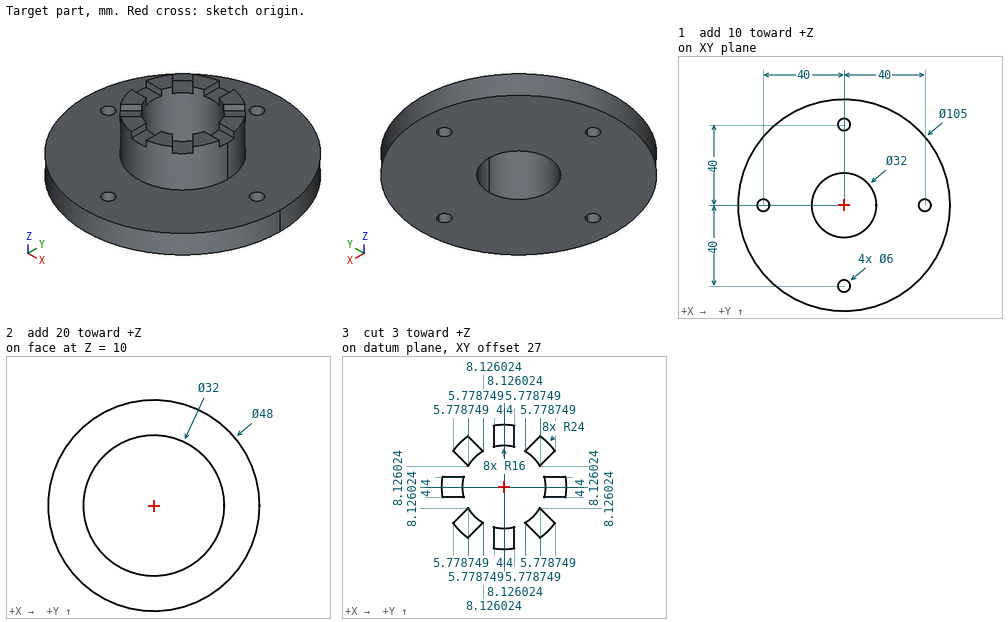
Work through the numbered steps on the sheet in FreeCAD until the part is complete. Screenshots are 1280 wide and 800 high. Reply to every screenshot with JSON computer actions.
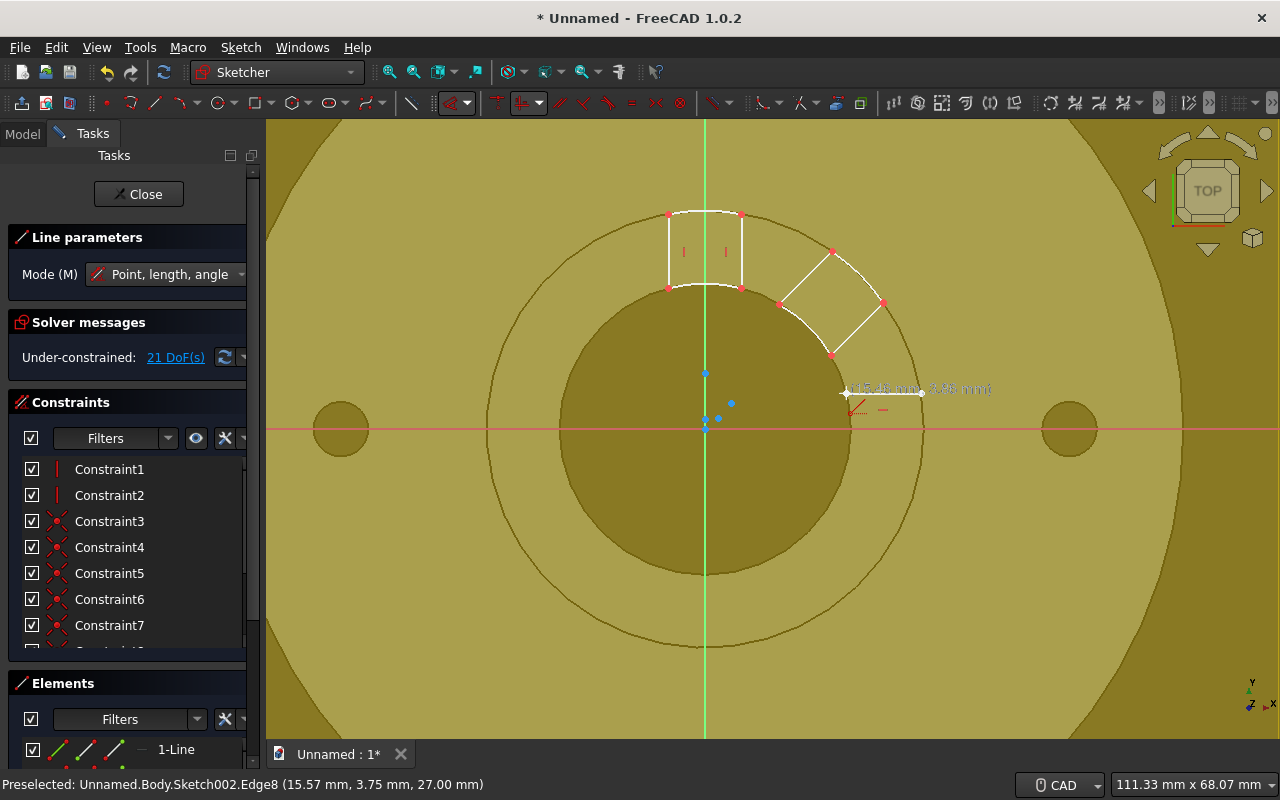
{"action": "left_click", "coordinate": [846, 466]}
{"action": "left_click", "coordinate": [921, 466]}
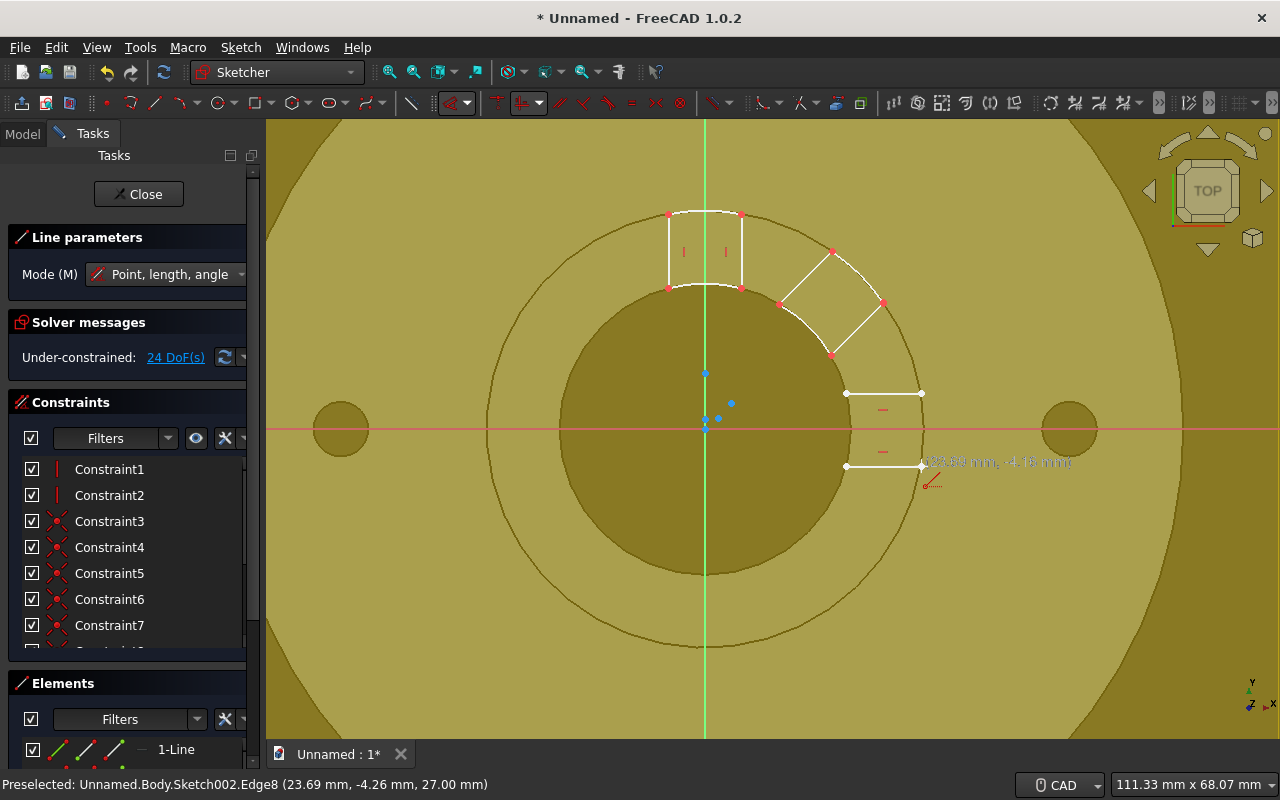
{"action": "left_click", "coordinate": [180, 104]}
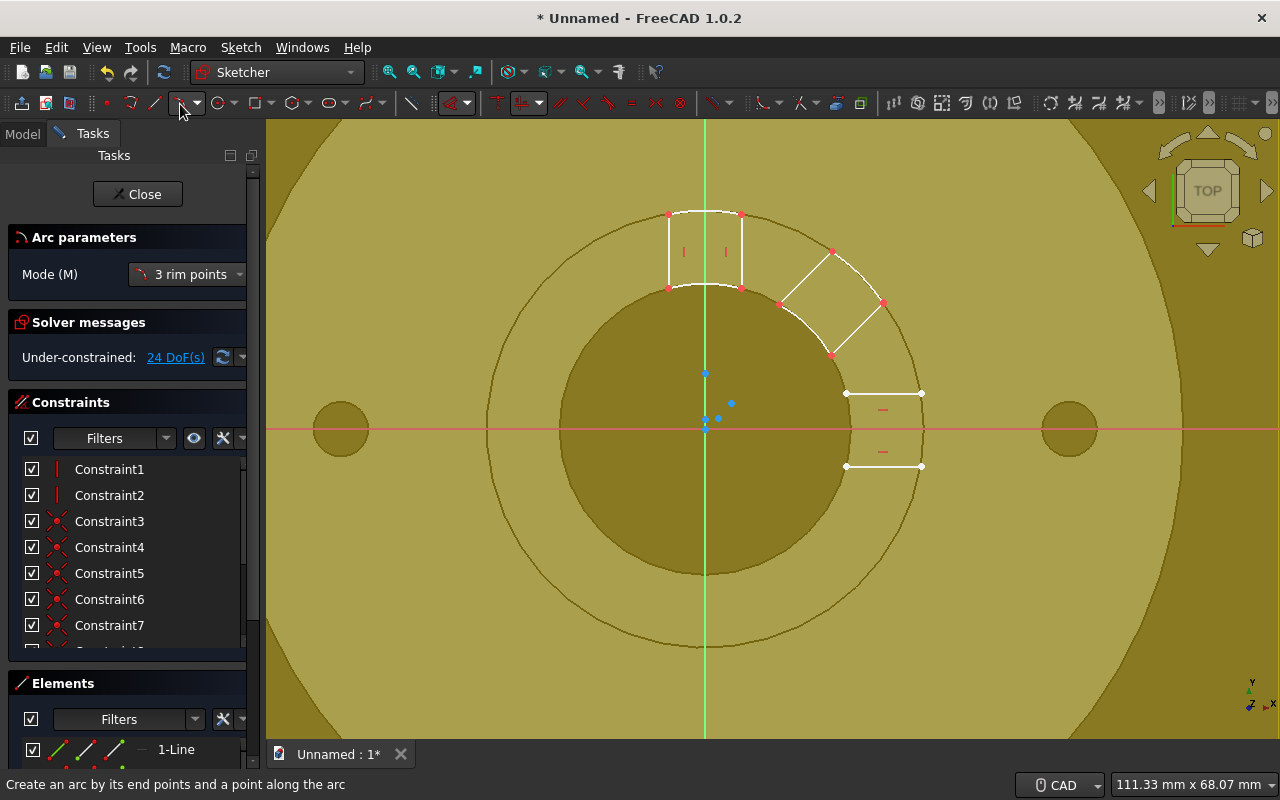
{"action": "left_click", "coordinate": [846, 394]}
{"action": "left_click", "coordinate": [846, 467]}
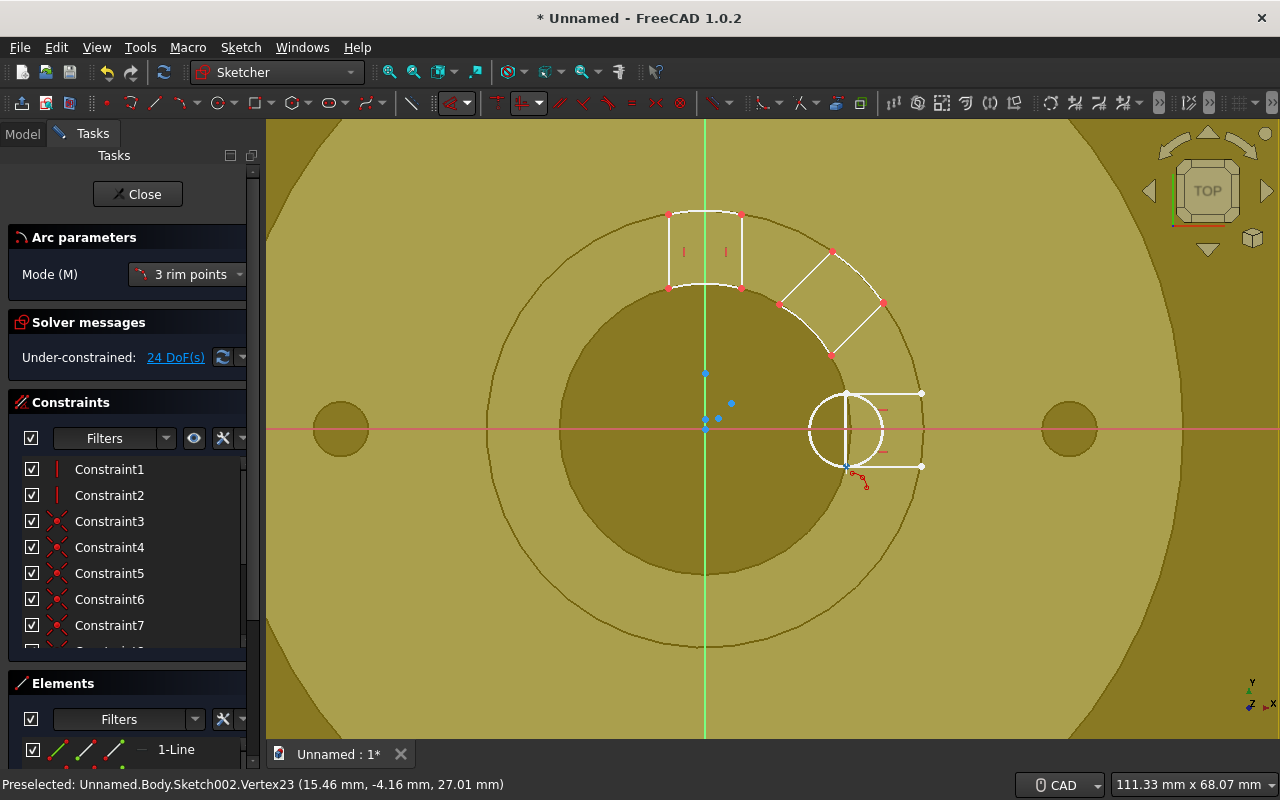
{"action": "scroll", "coordinate": [851, 437], "scroll_direction": "up", "scroll_amount": 7}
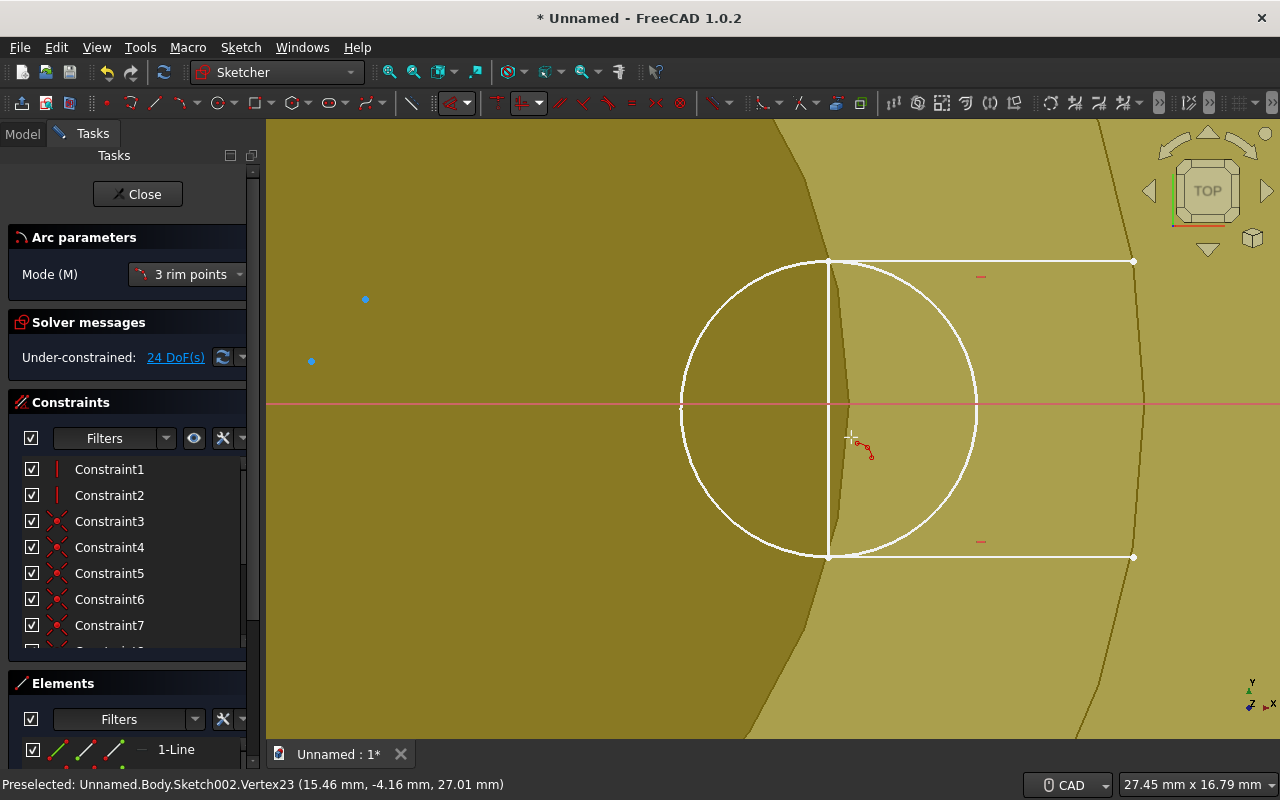
{"action": "left_click", "coordinate": [848, 433]}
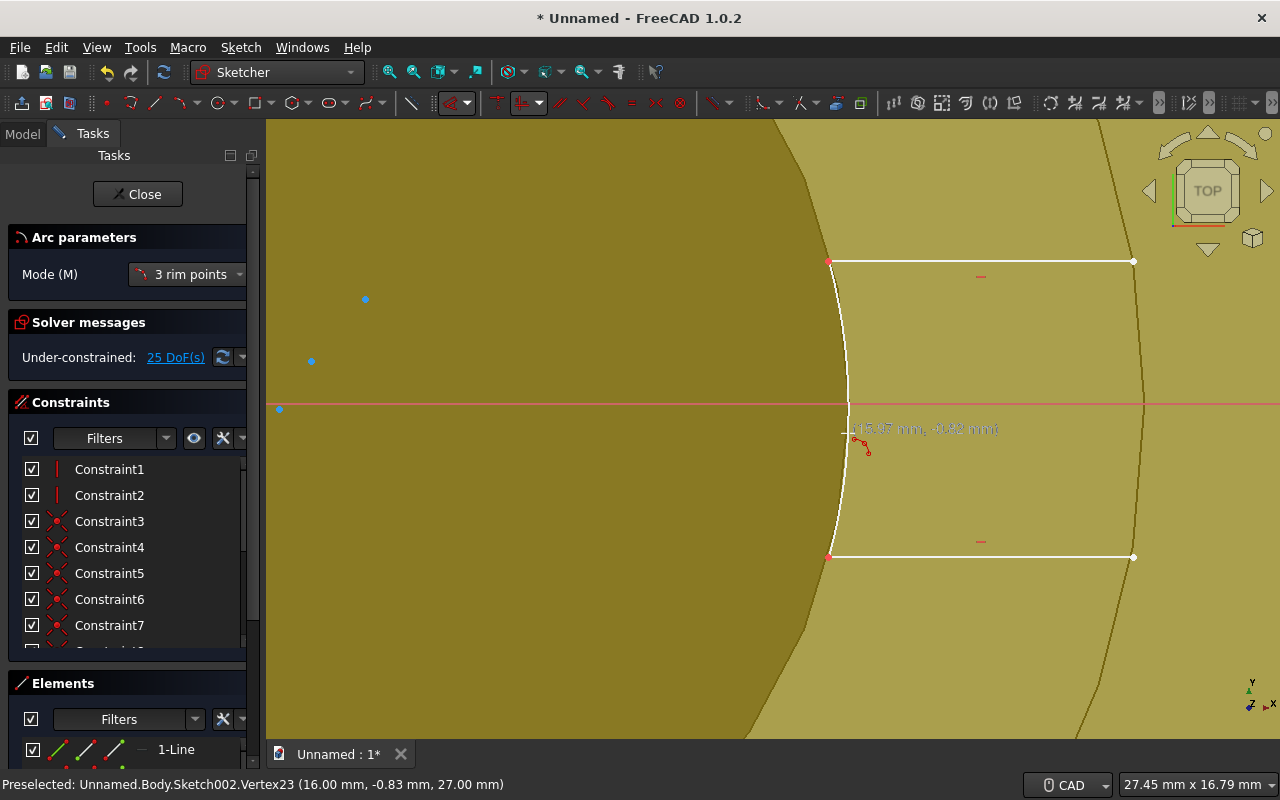
{"action": "scroll", "coordinate": [851, 437], "scroll_direction": "down", "scroll_amount": 7}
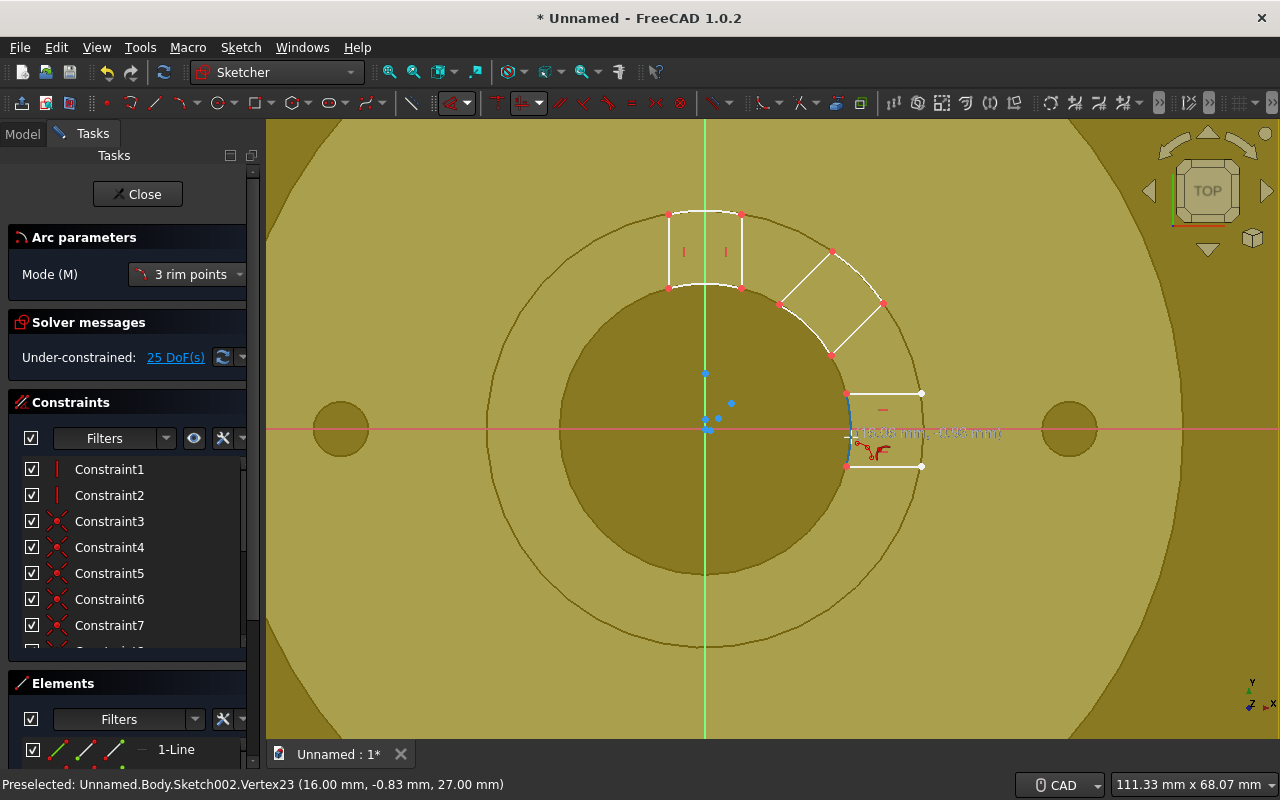
{"action": "left_click", "coordinate": [921, 467]}
{"action": "left_click", "coordinate": [921, 394]}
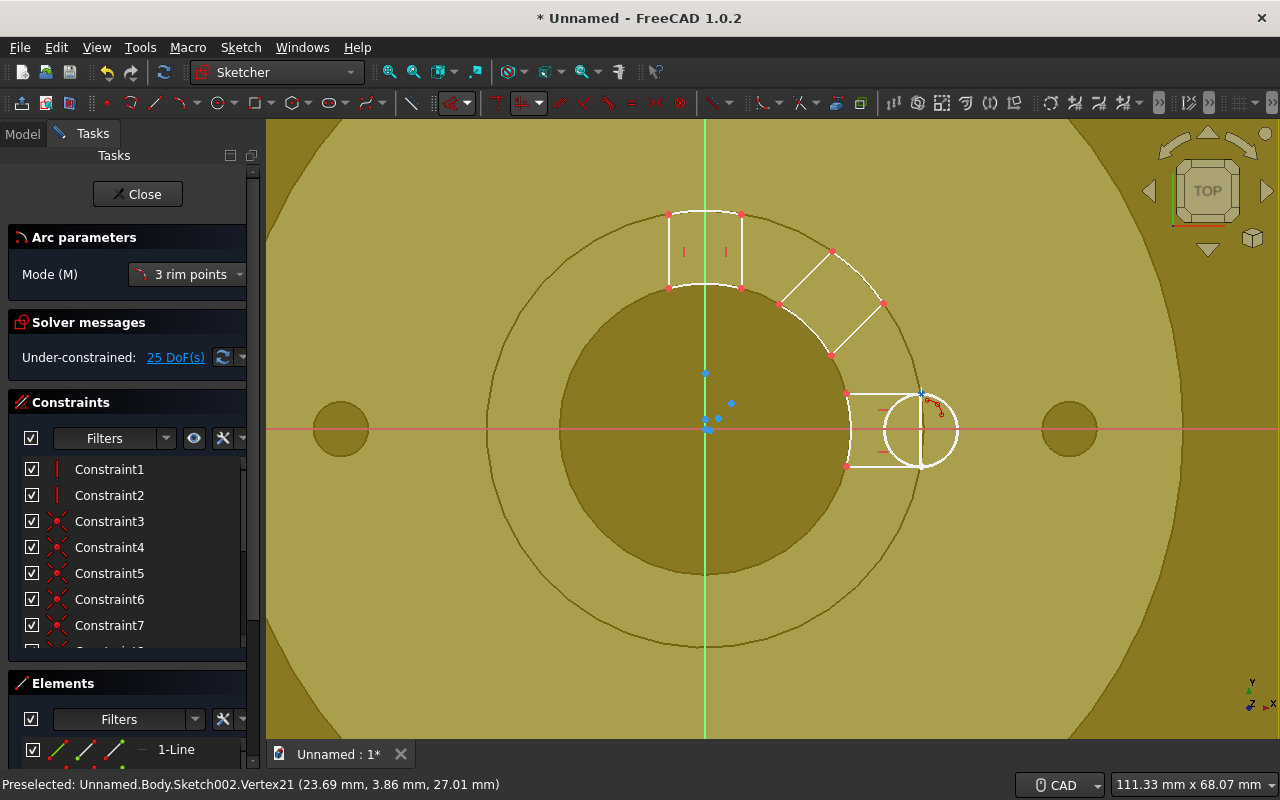
{"action": "scroll", "coordinate": [924, 436], "scroll_direction": "up", "scroll_amount": 9}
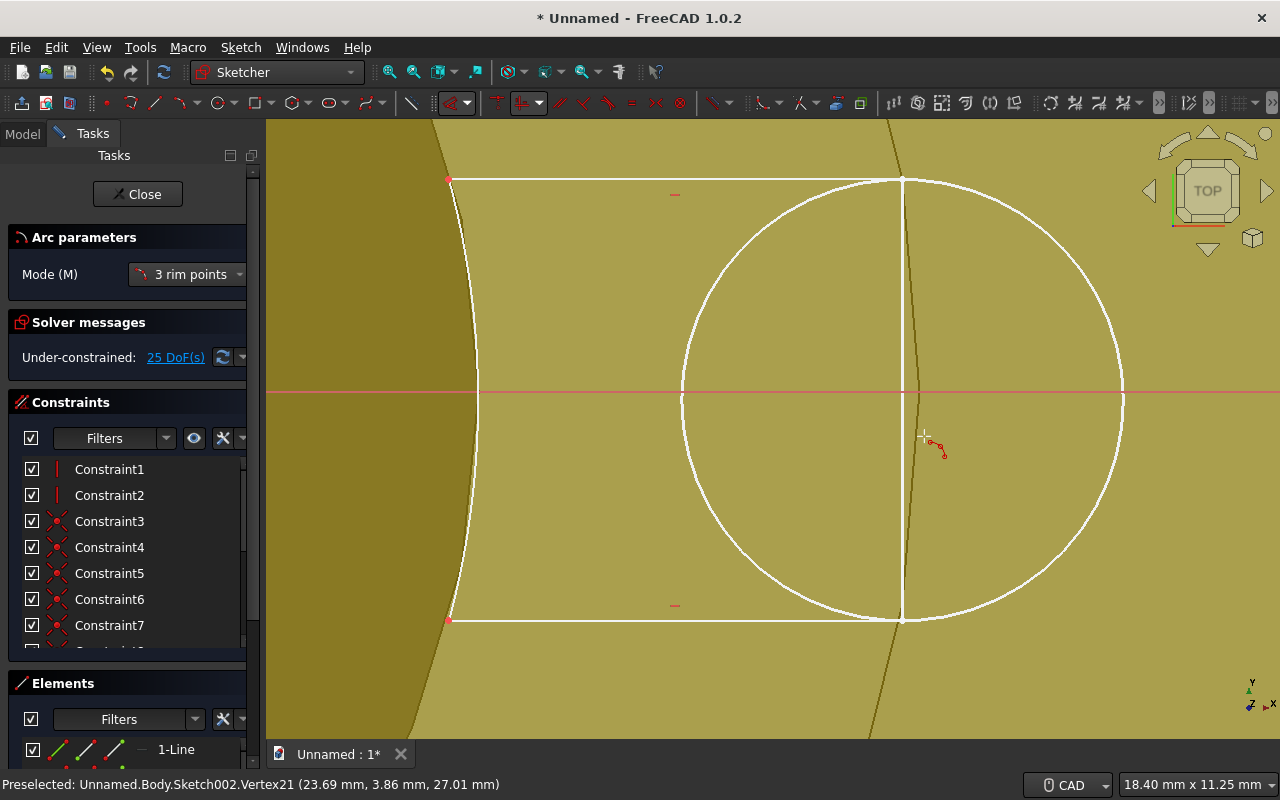
{"action": "left_click", "coordinate": [919, 436]}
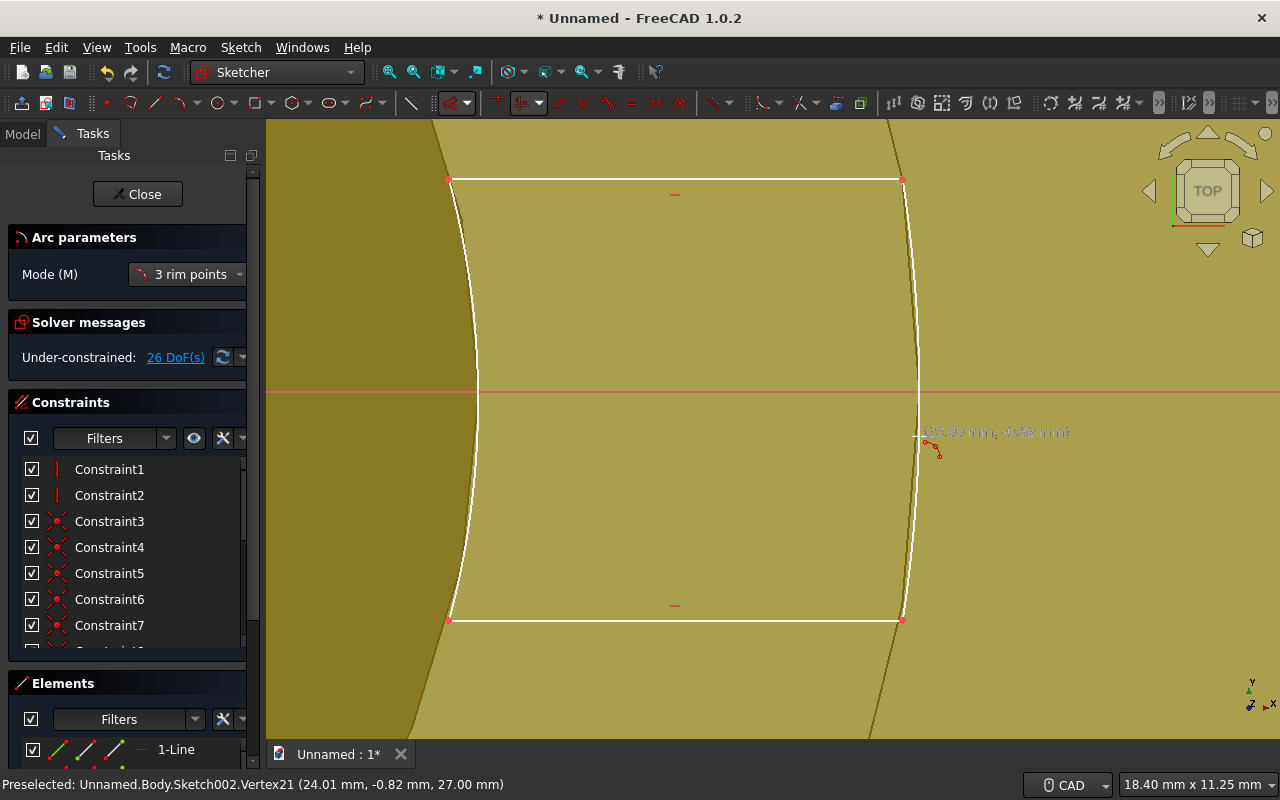
{"action": "left_click", "coordinate": [156, 104]}